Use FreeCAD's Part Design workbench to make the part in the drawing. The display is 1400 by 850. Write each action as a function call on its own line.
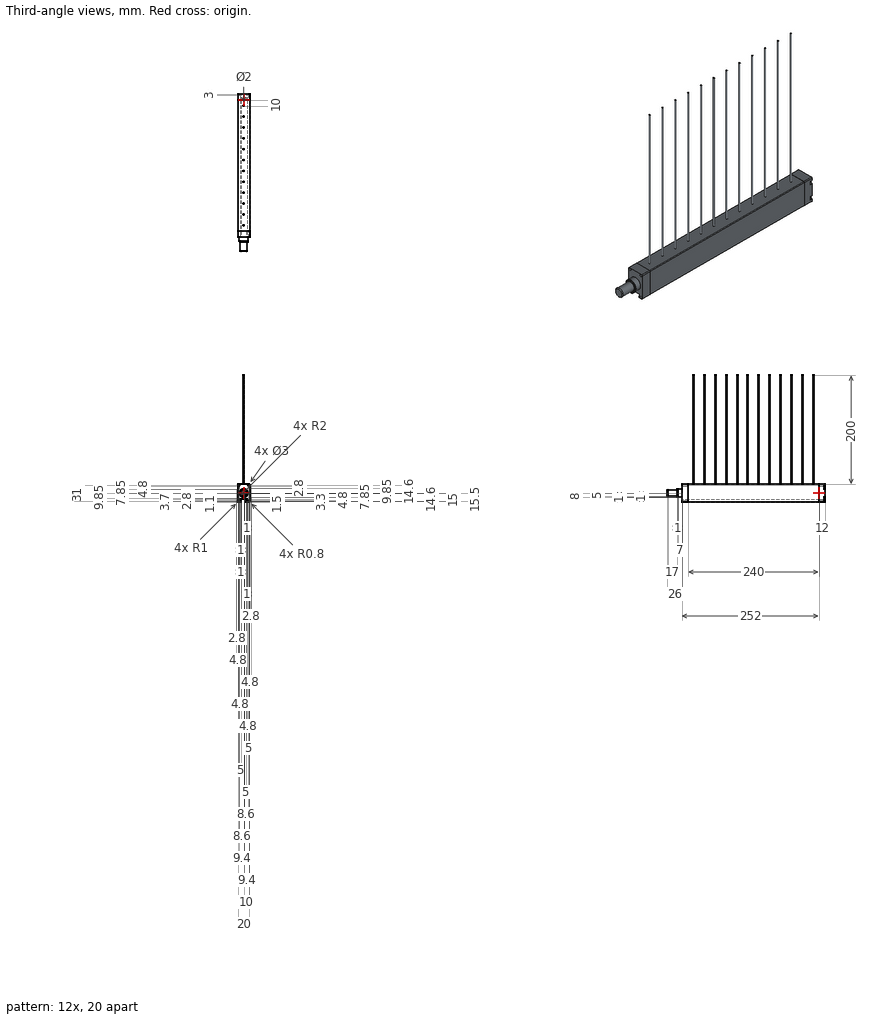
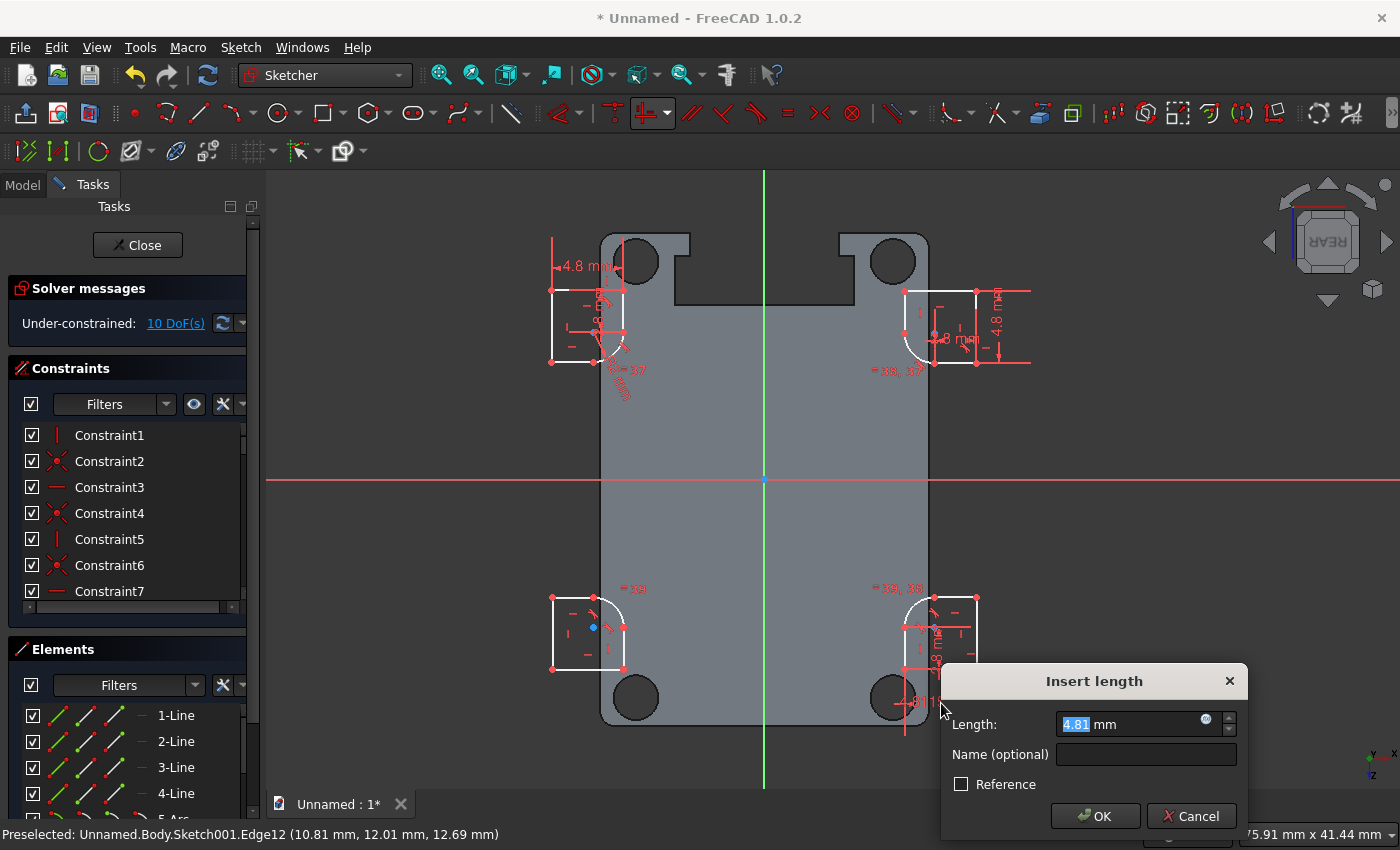
text(4.8)
key(Return)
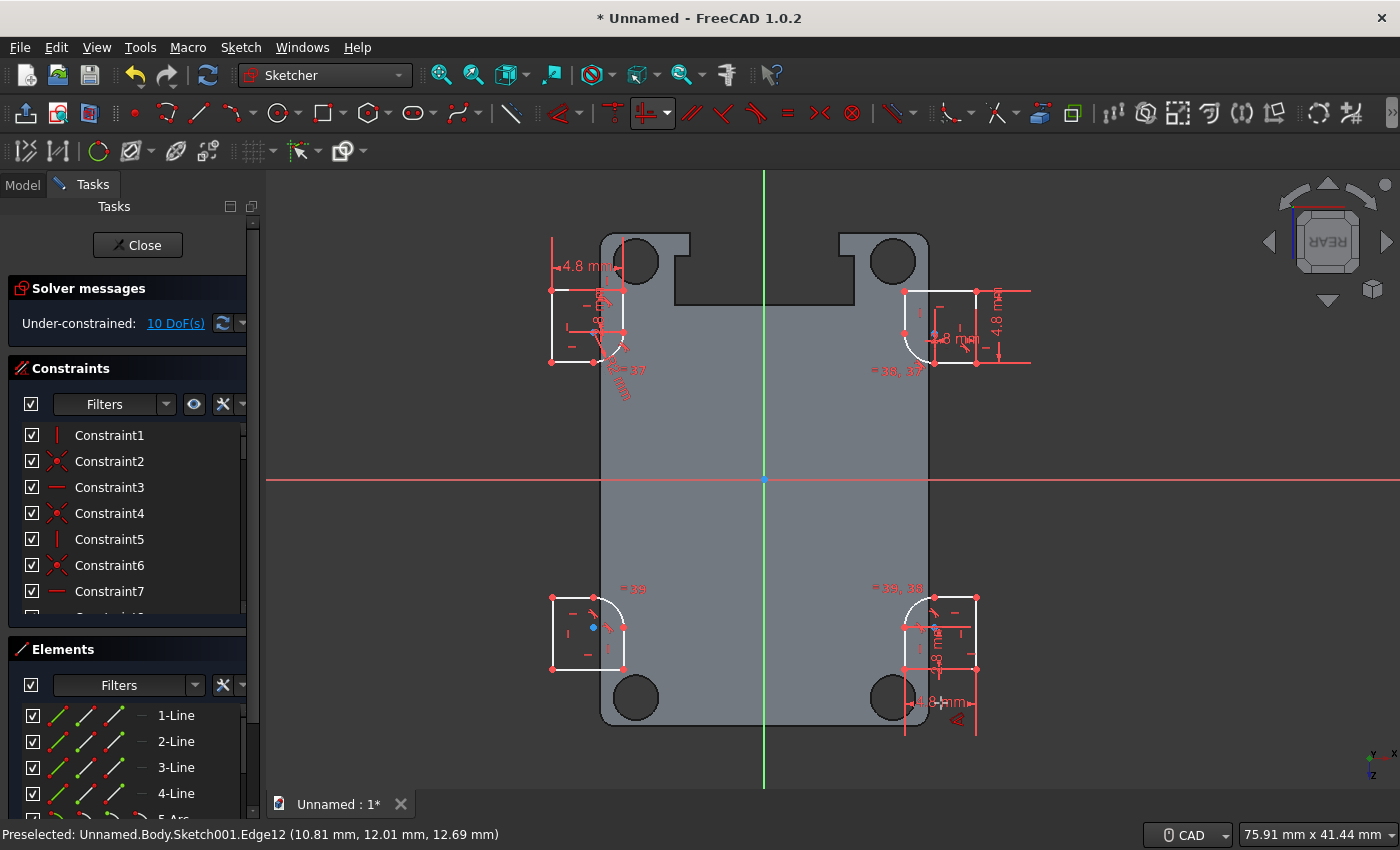
click(582, 598)
click(573, 632)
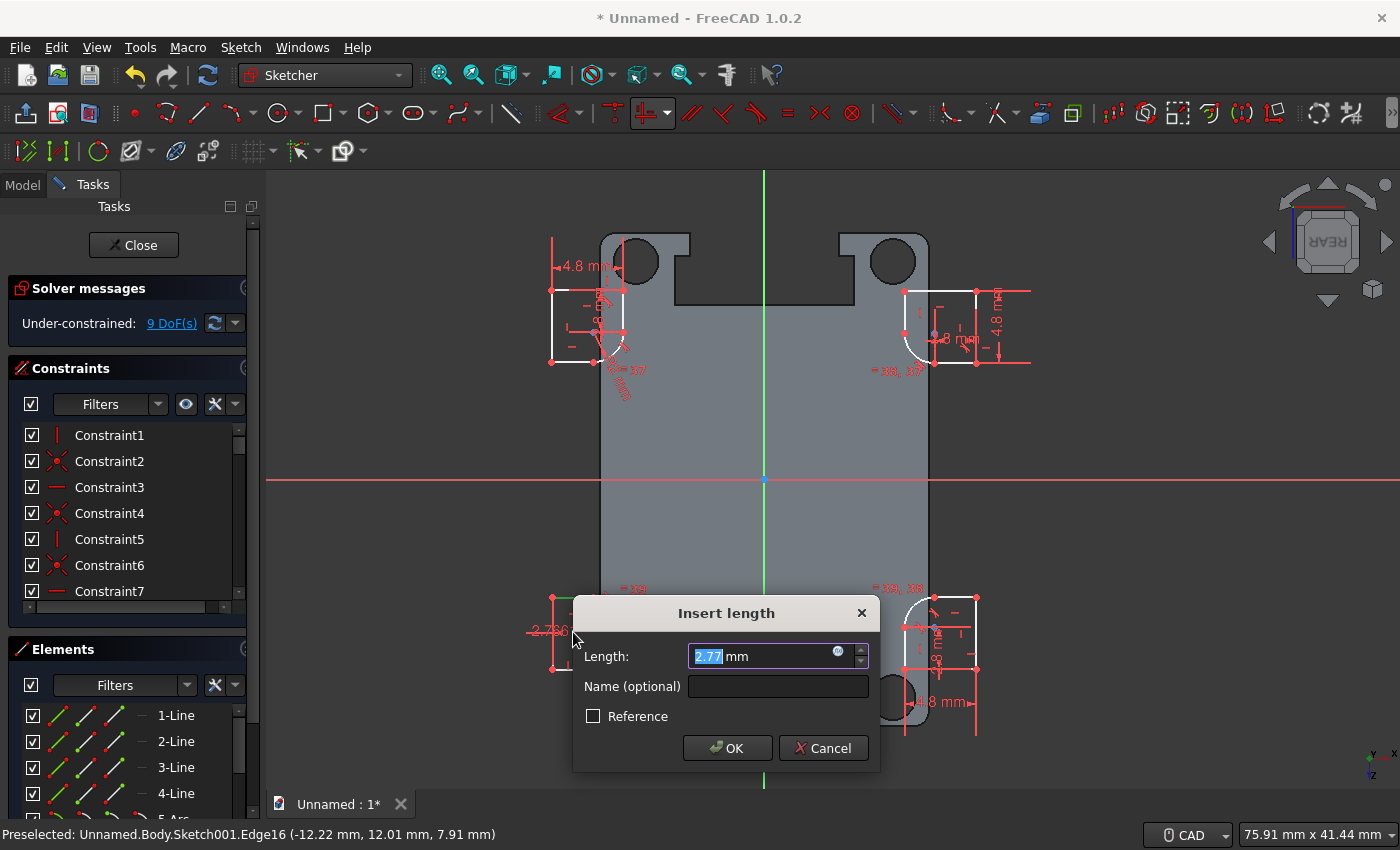
text(2.8)
key(Return)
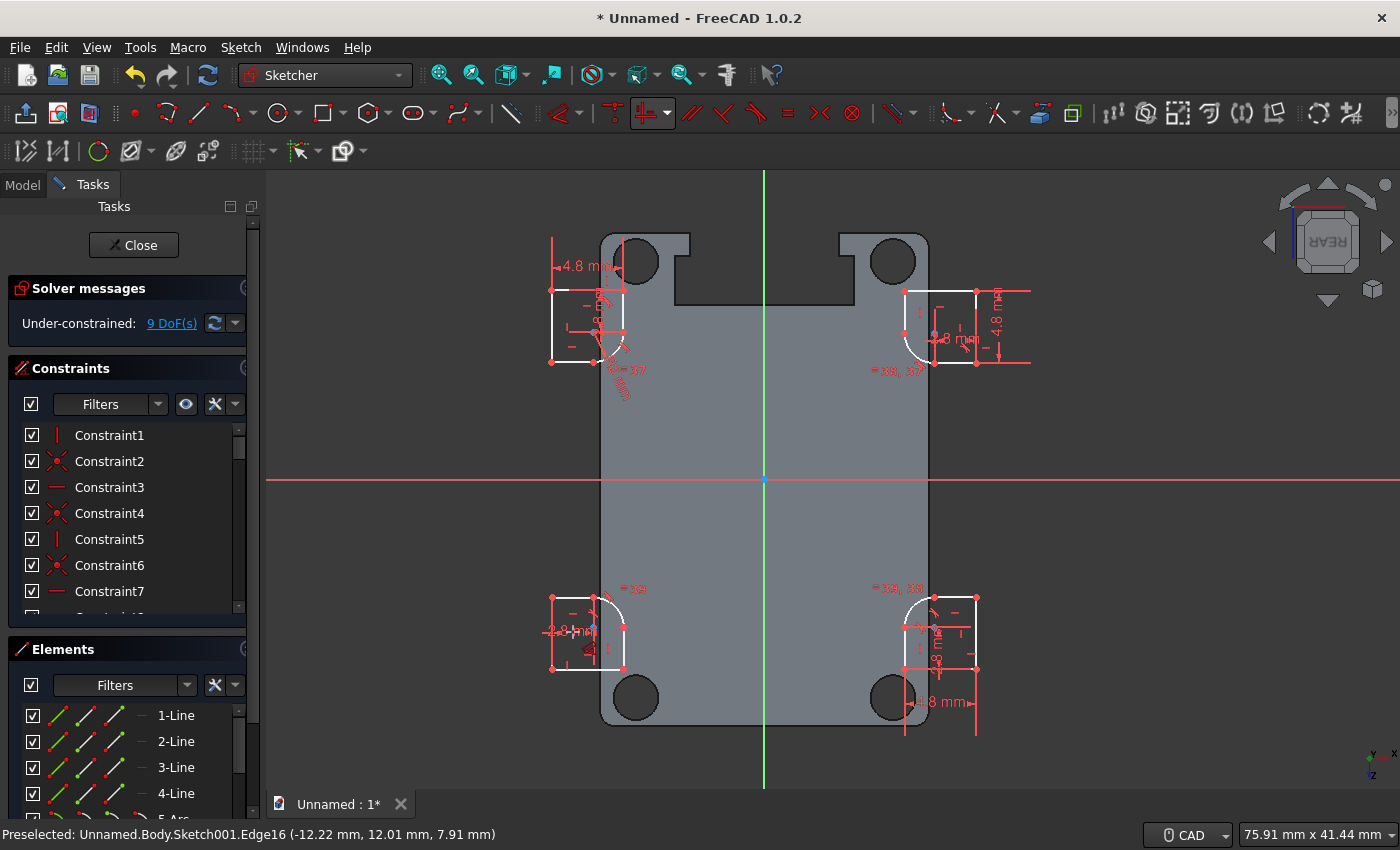
click(552, 619)
click(518, 609)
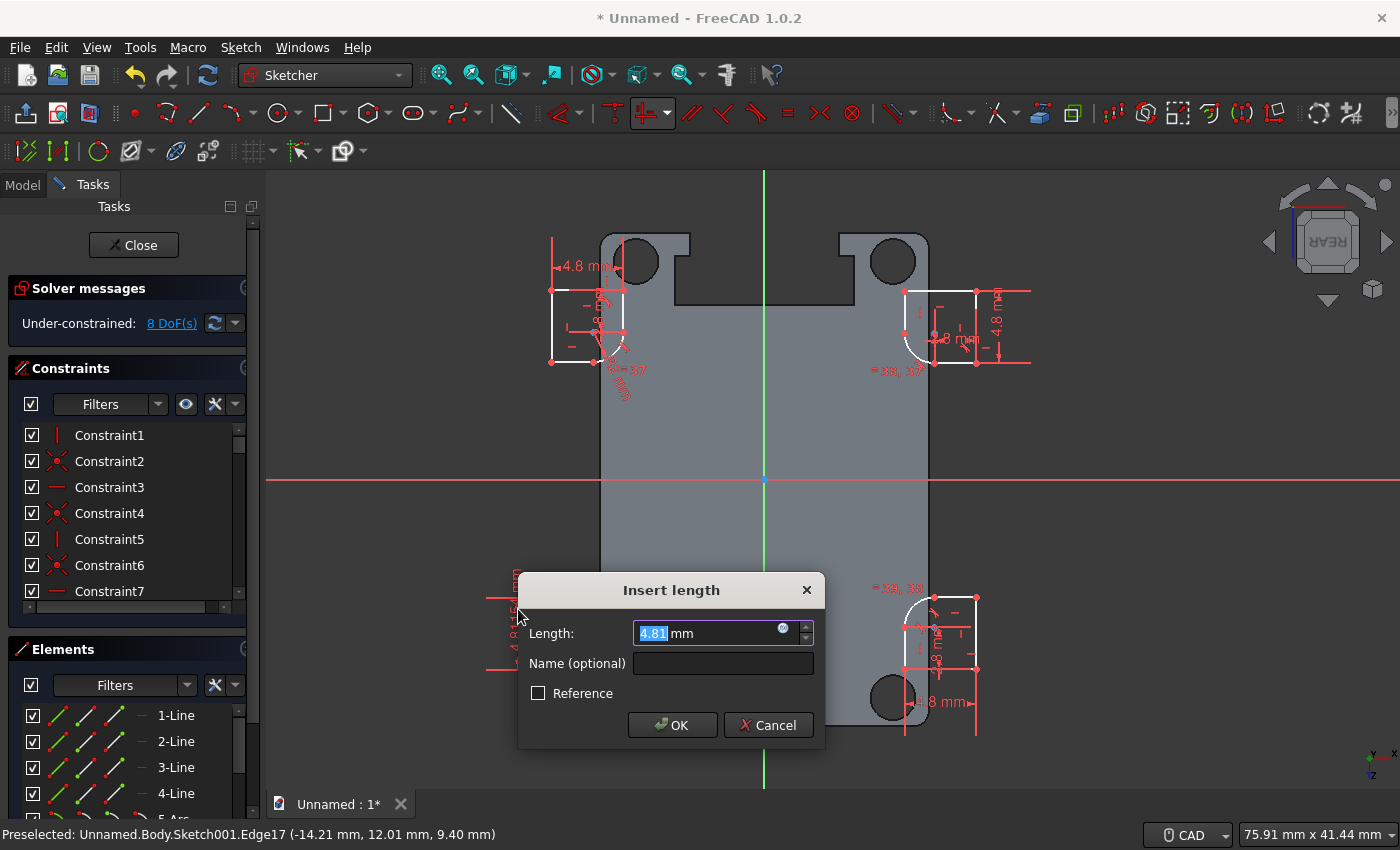
text(4.8)
key(Return)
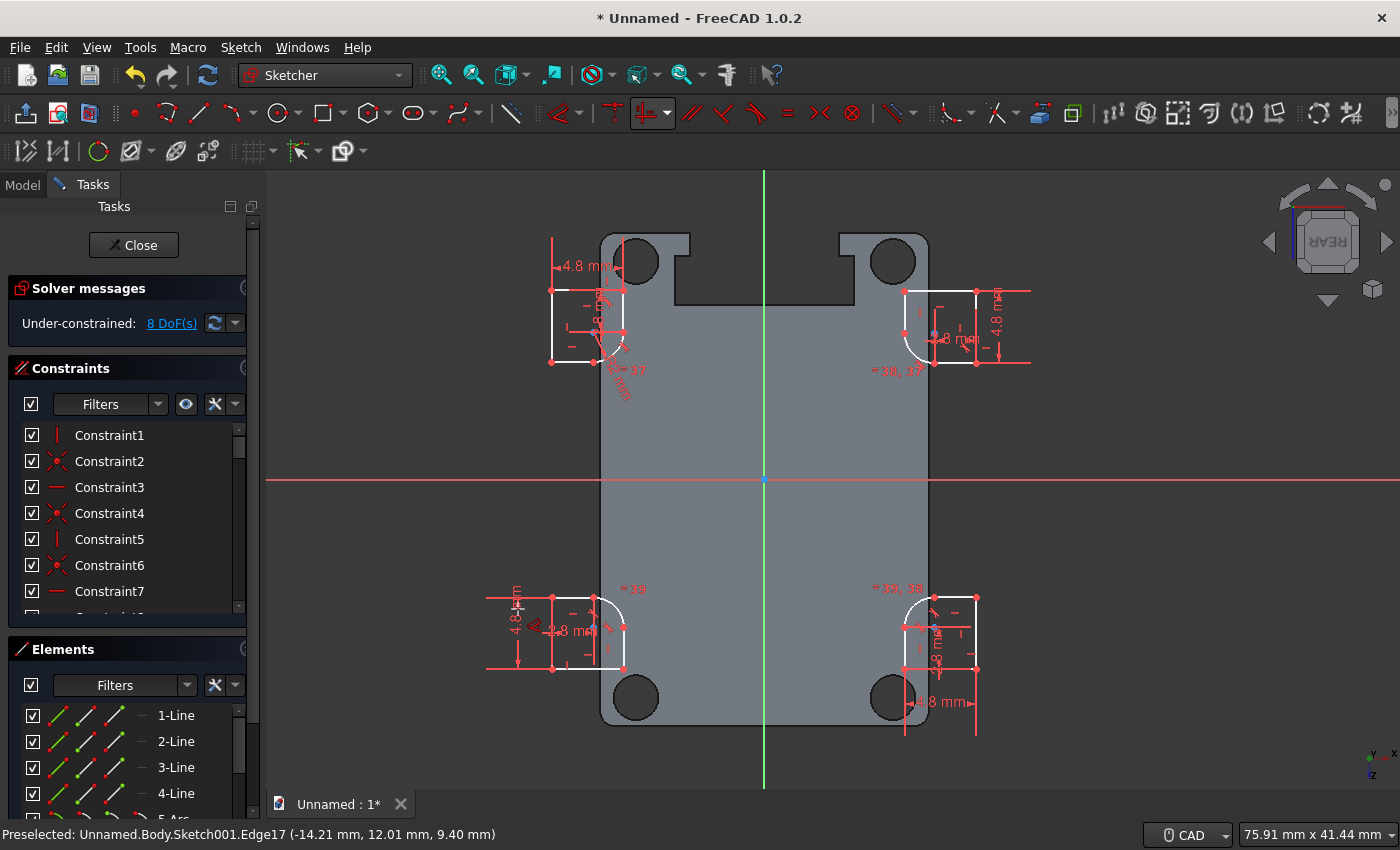
click(623, 332)
click(694, 298)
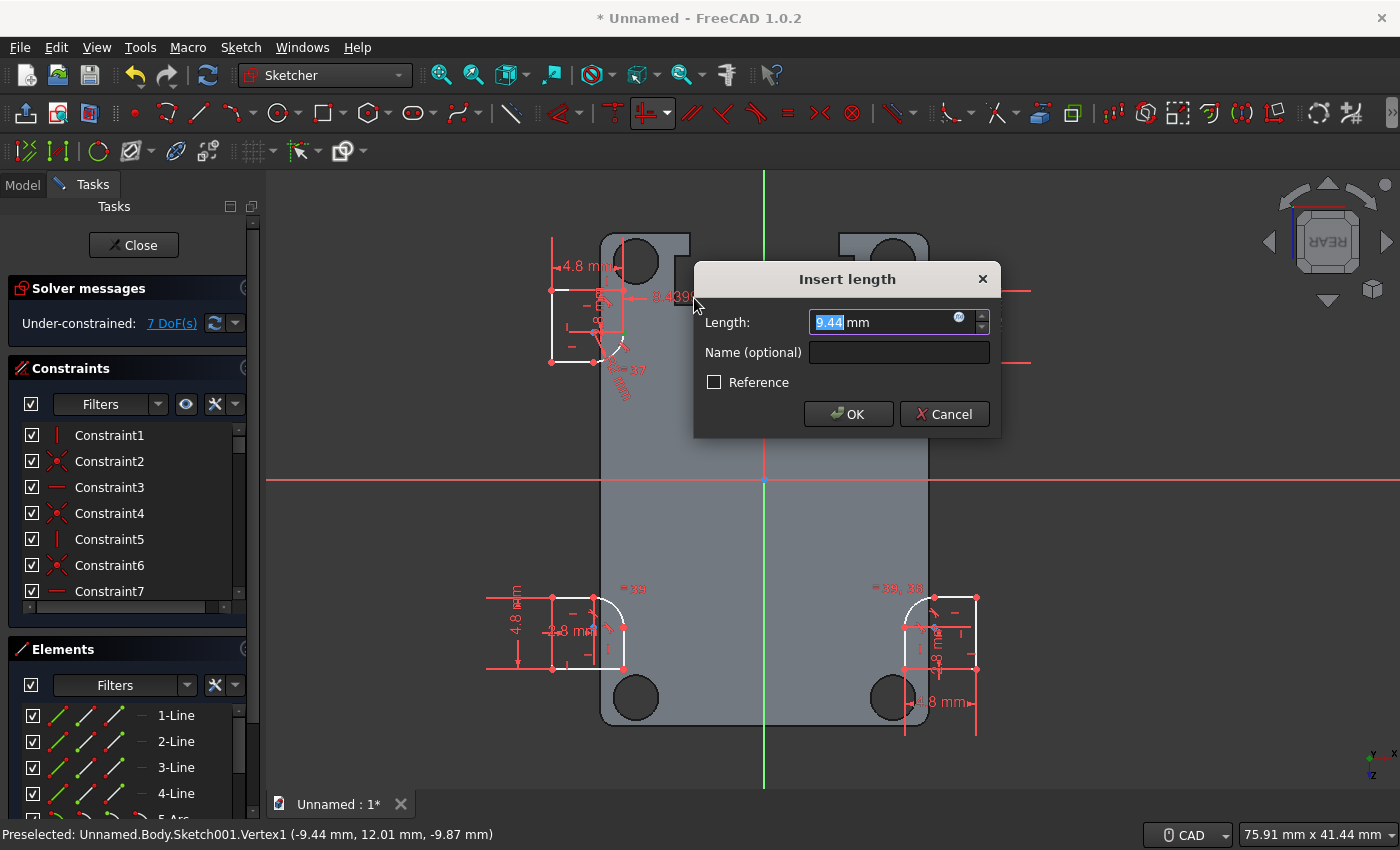
text(9.4)
key(Return)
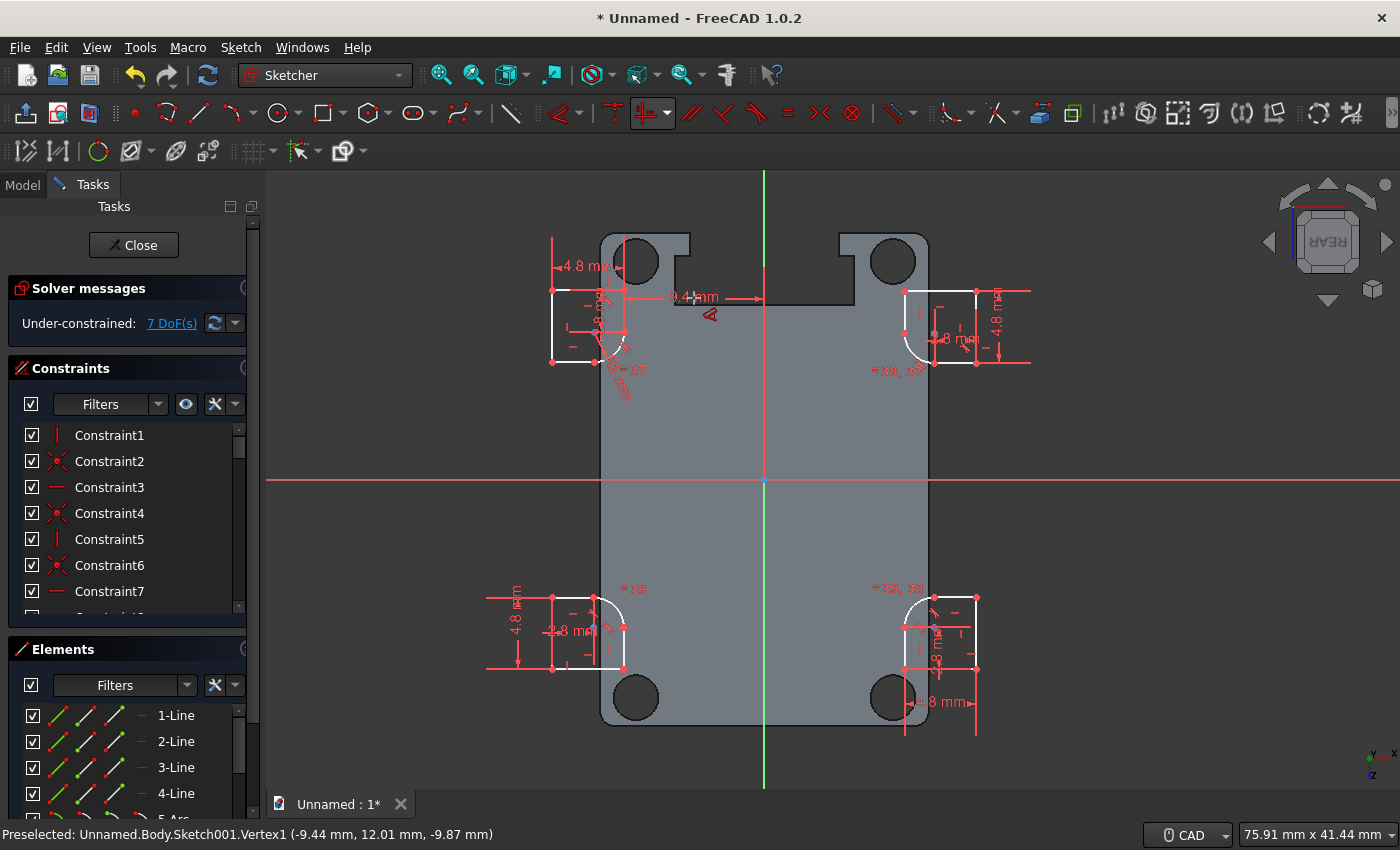
click(905, 291)
click(835, 257)